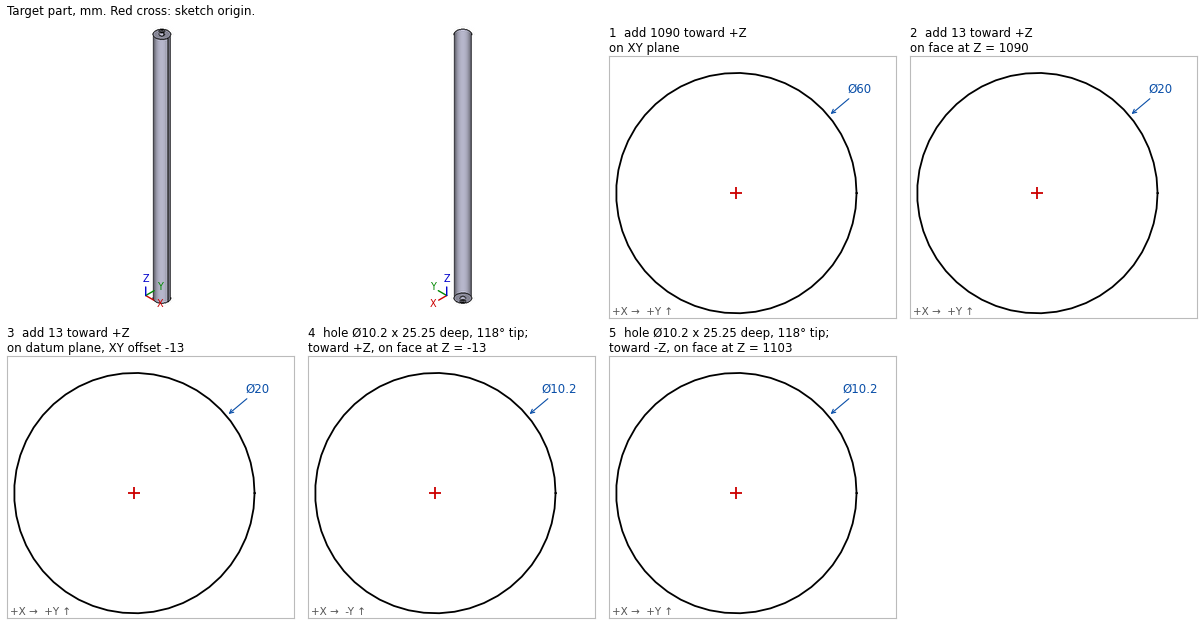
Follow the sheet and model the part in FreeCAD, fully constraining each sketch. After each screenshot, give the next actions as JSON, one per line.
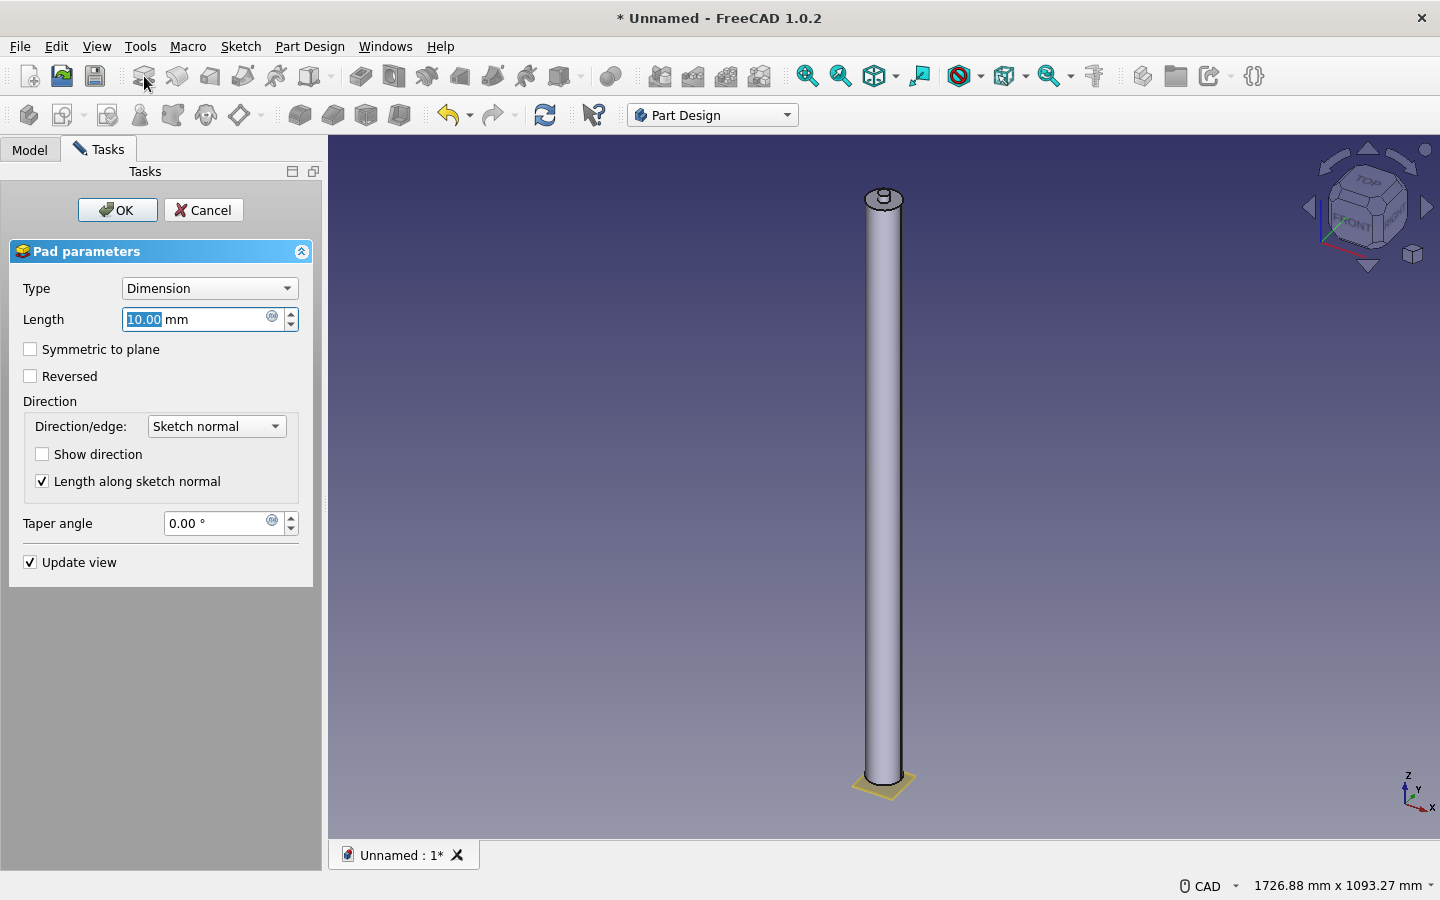
{"action": "type", "text": "13"}
{"action": "key", "text": "Tab"}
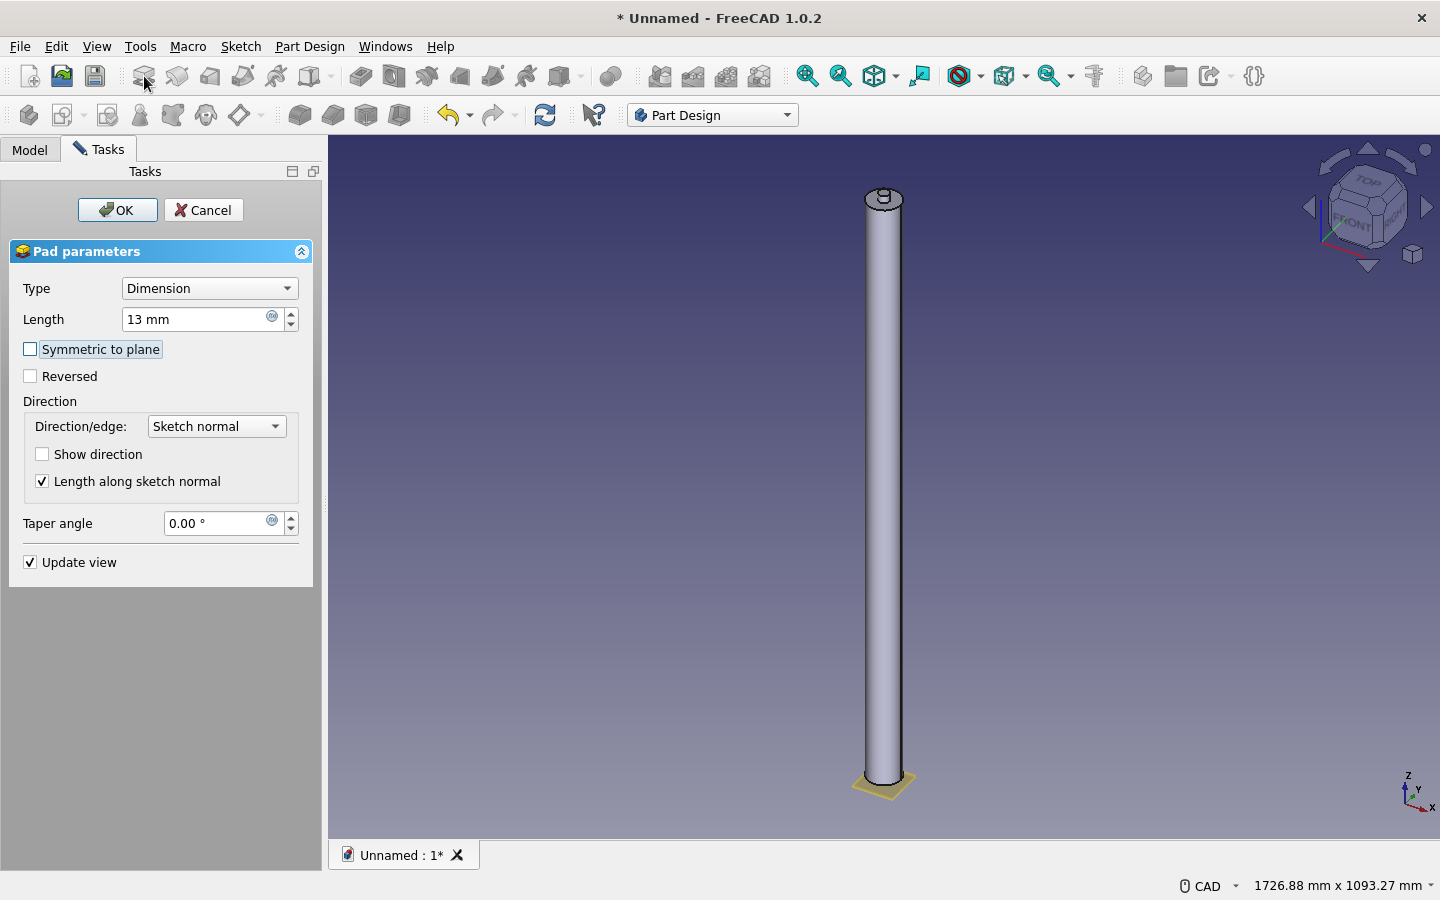
{"action": "left_click", "coordinate": [118, 210]}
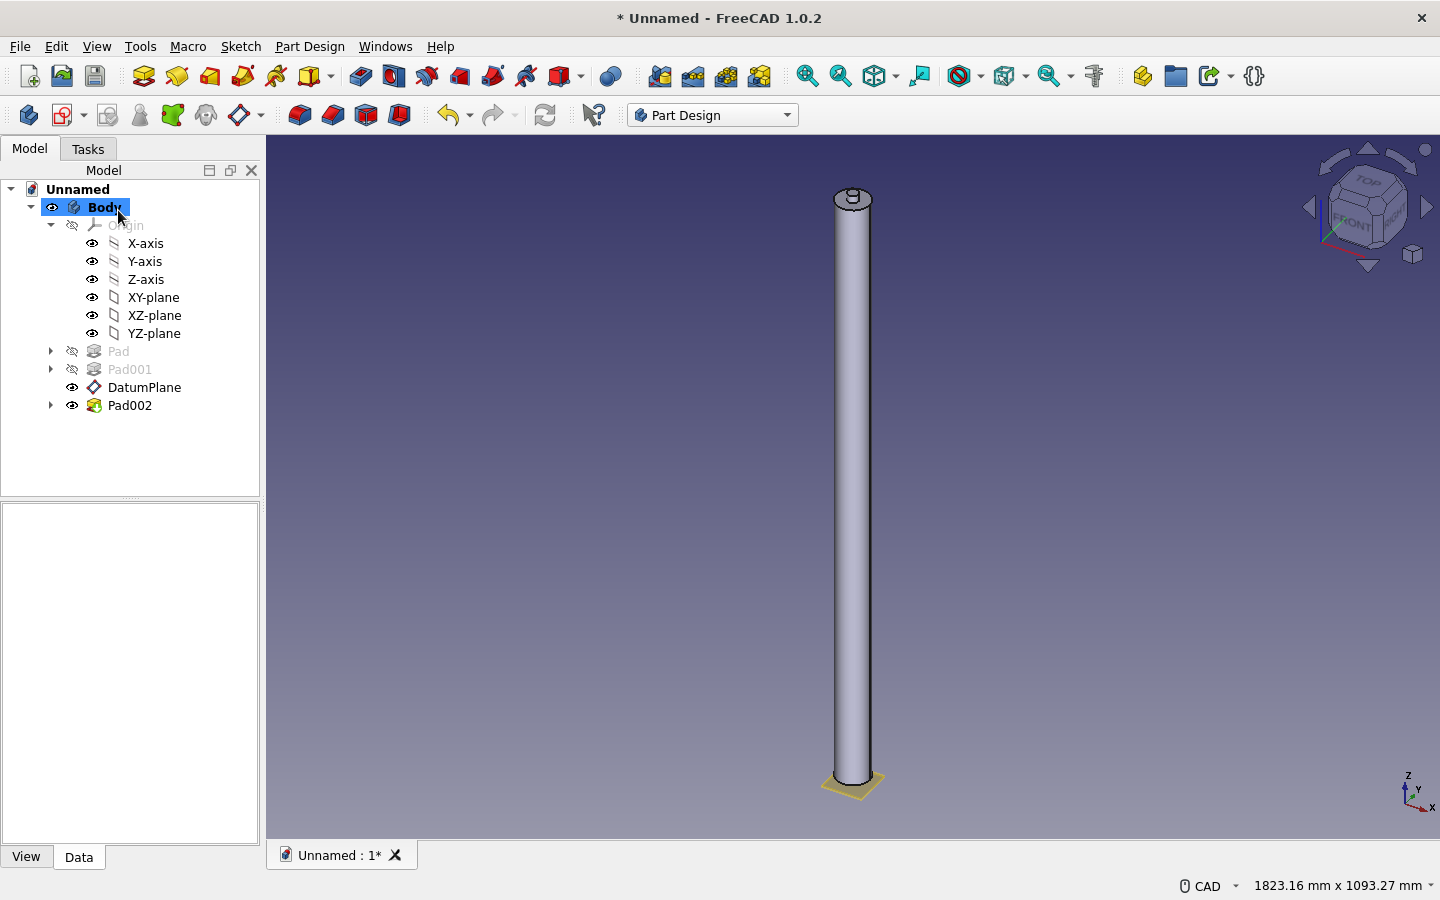
{"action": "left_click", "coordinate": [117, 387]}
{"action": "key", "text": "space"}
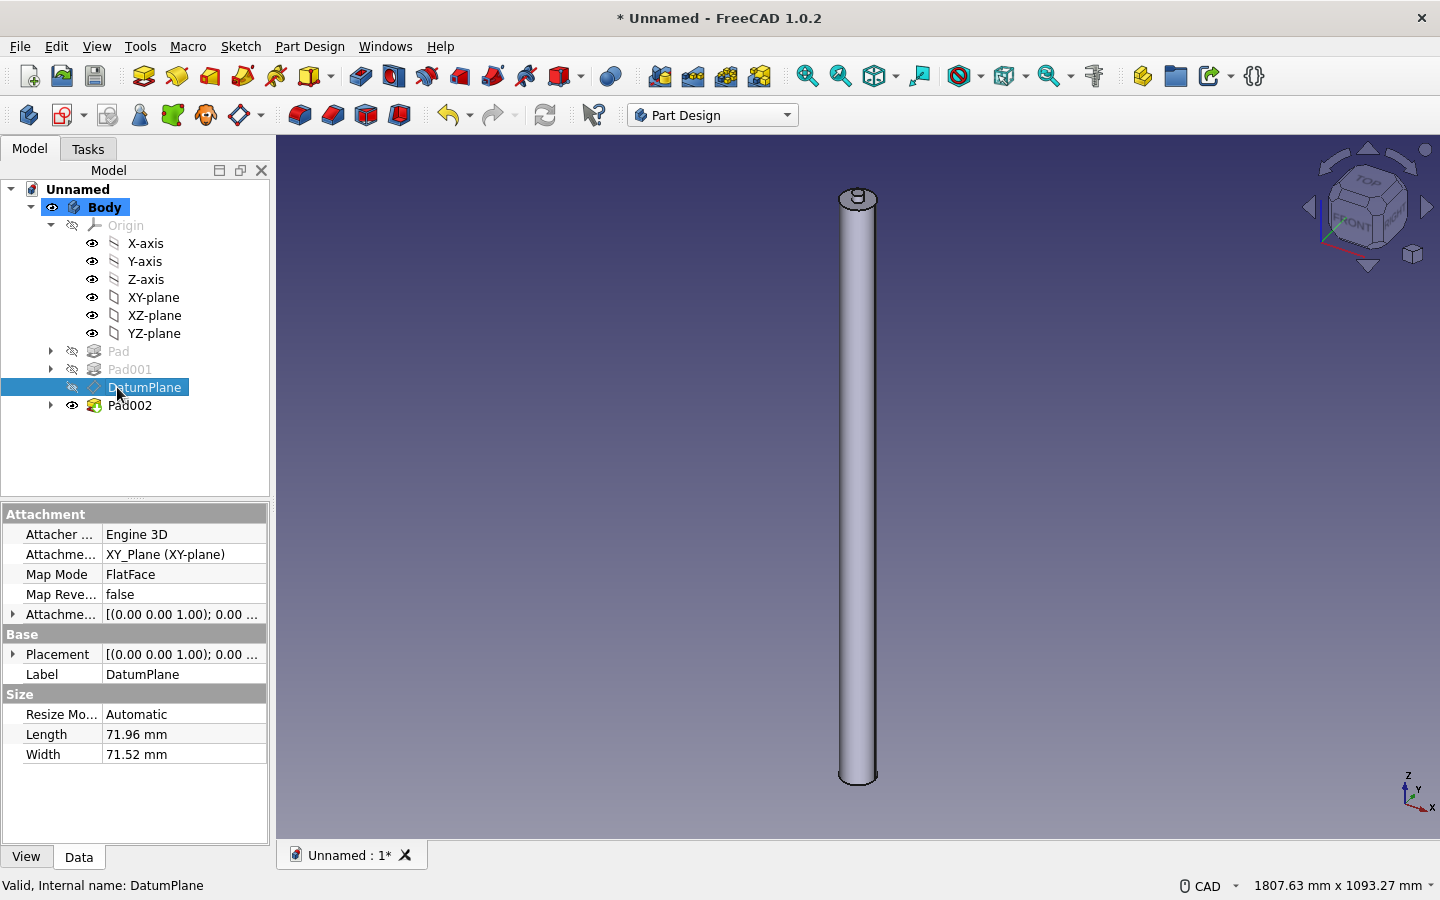
{"action": "key", "text": "5"}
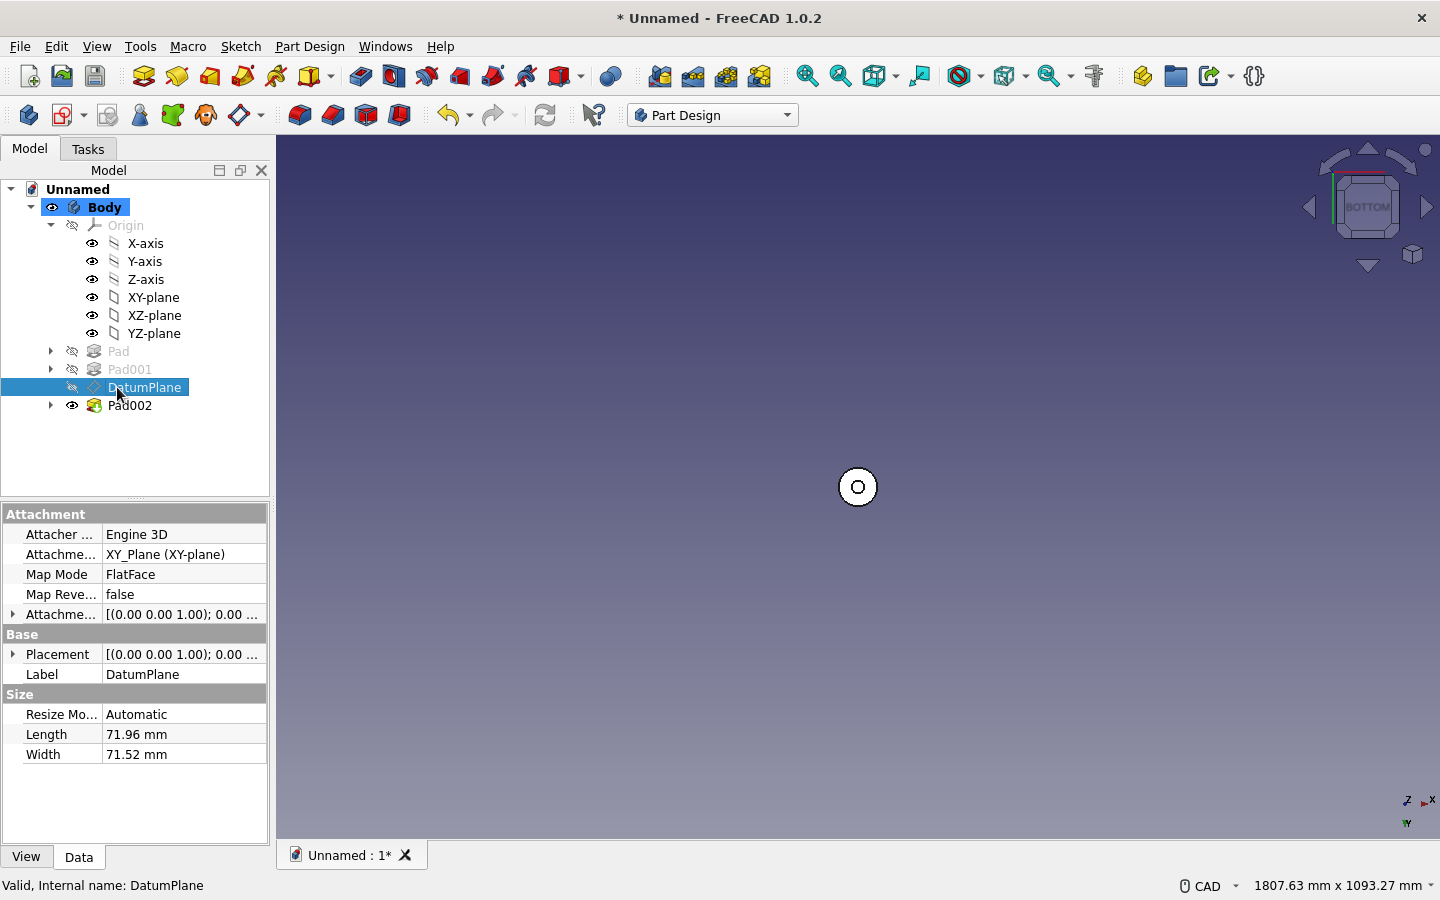
{"action": "key", "text": "v f"}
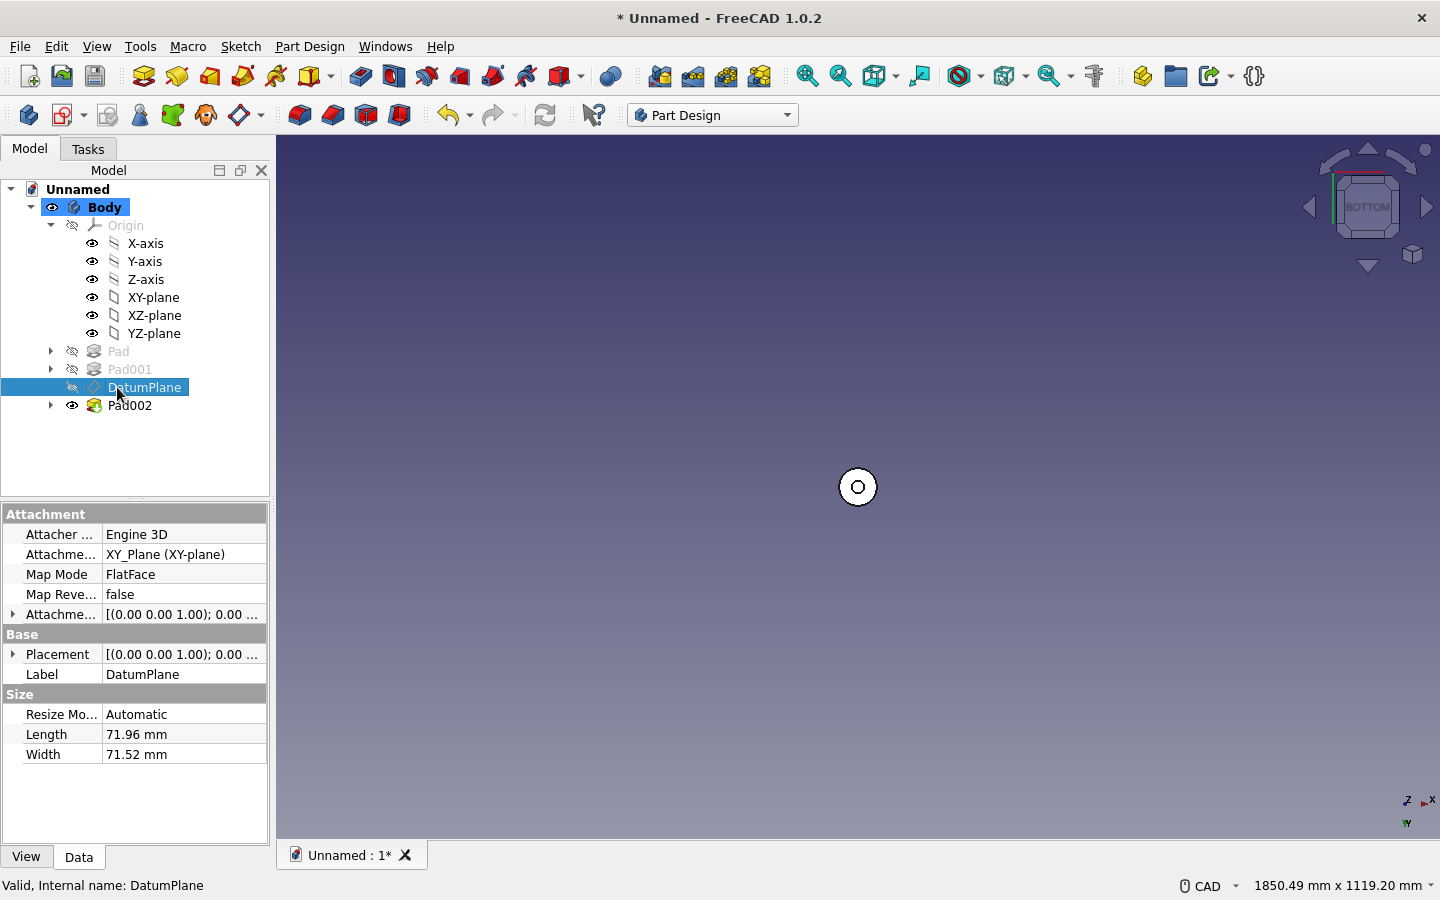
{"action": "scroll", "coordinate": [858, 486], "scroll_direction": "up", "scroll_amount": 4}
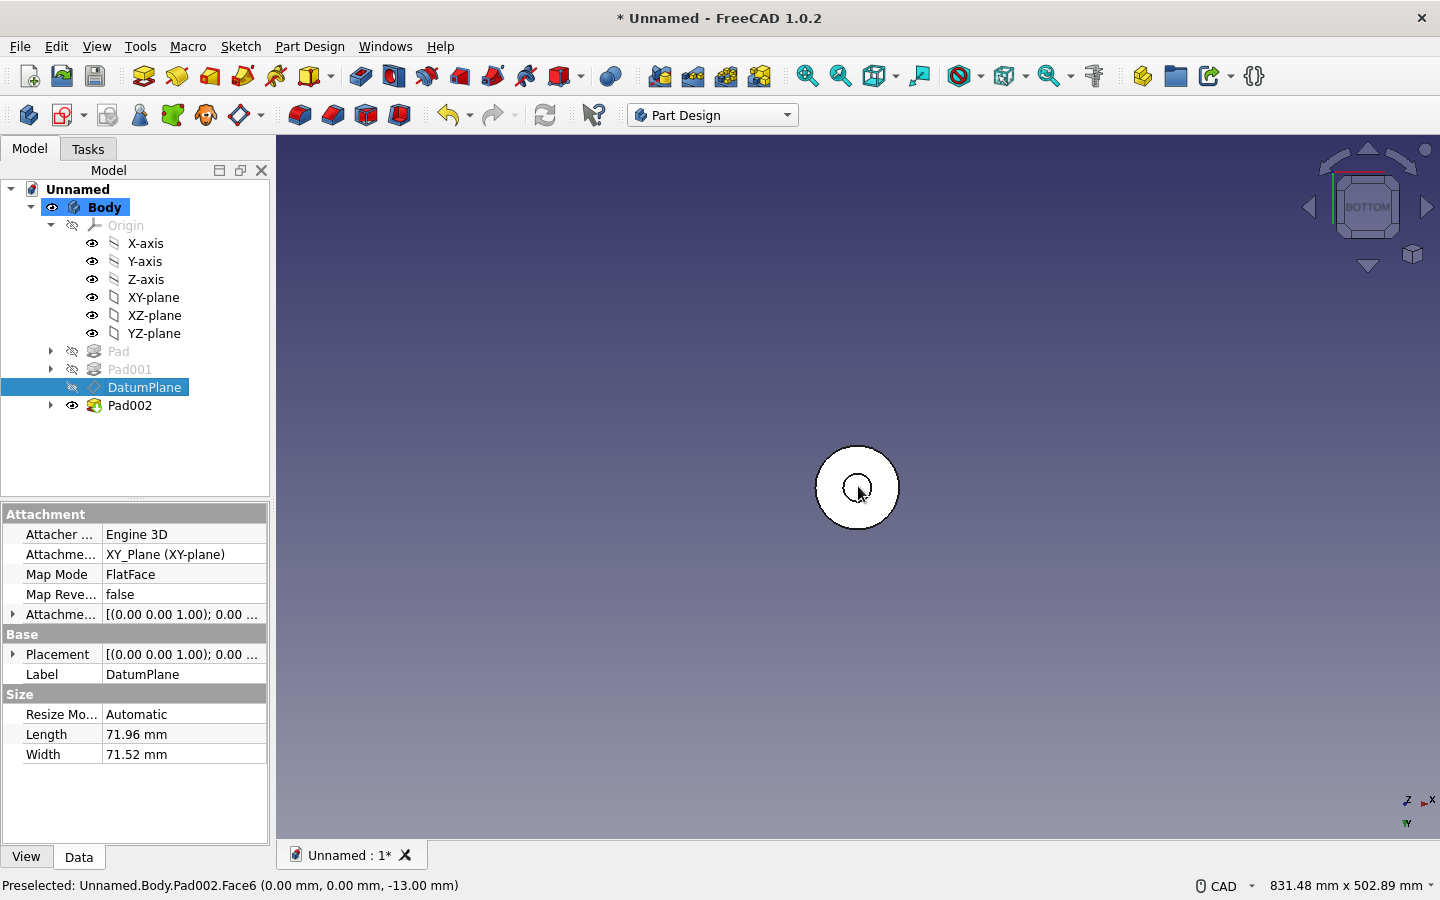
{"action": "left_click", "coordinate": [857, 487]}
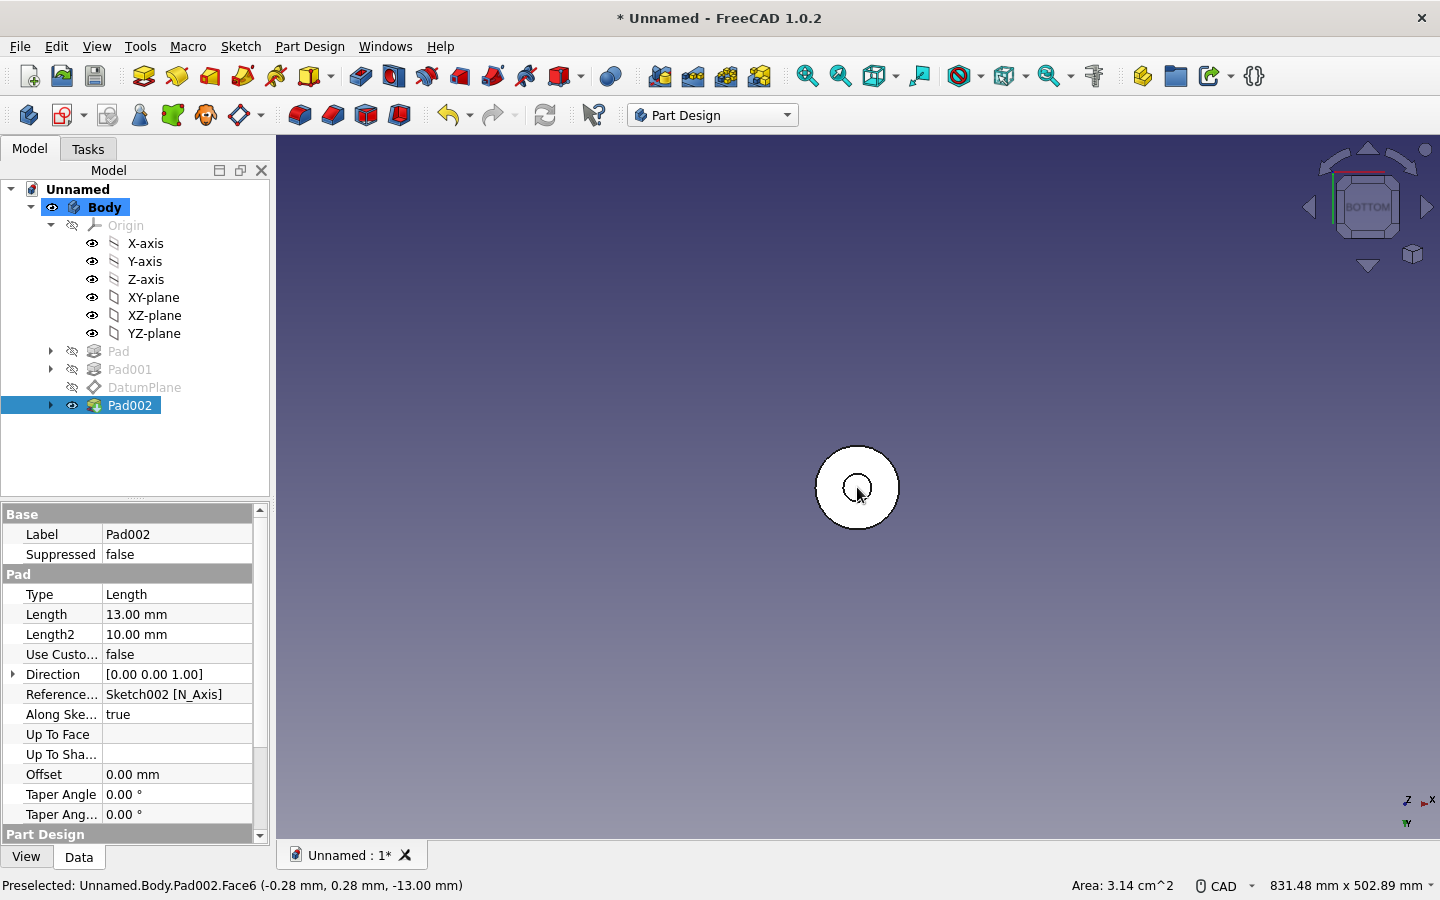
{"action": "left_click", "coordinate": [62, 116]}